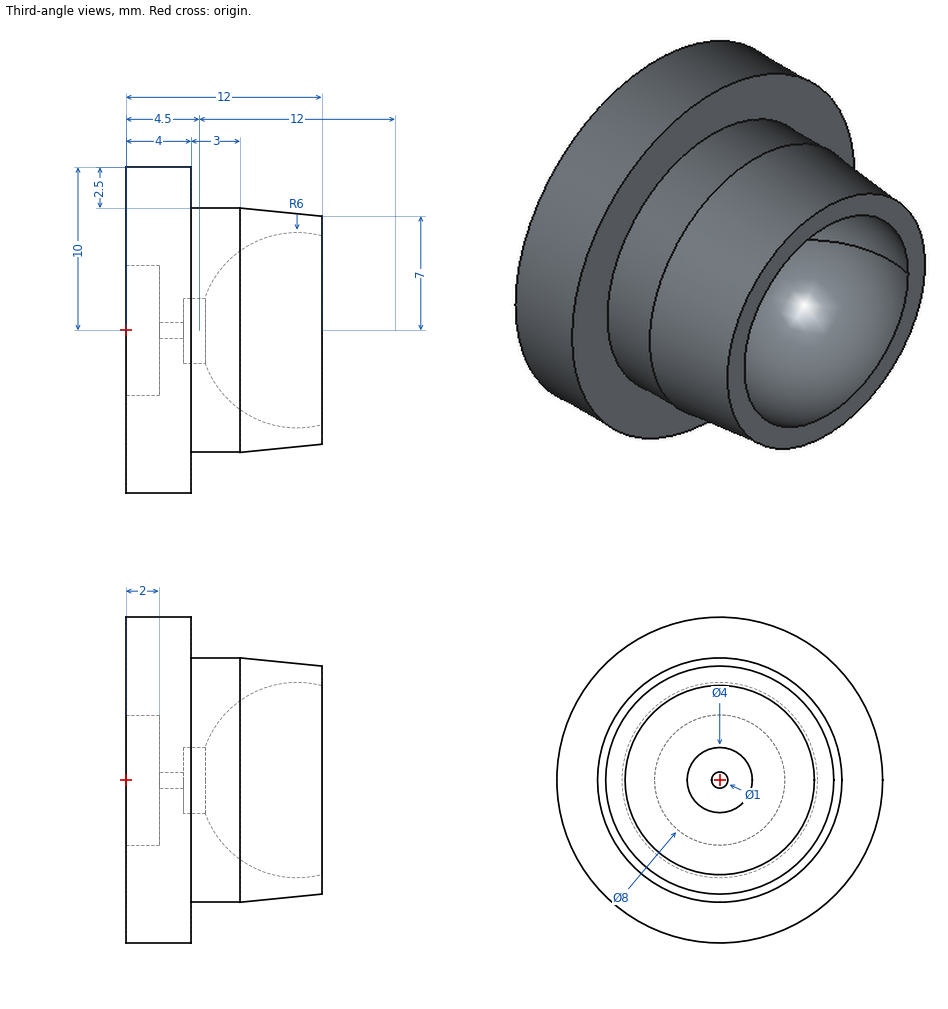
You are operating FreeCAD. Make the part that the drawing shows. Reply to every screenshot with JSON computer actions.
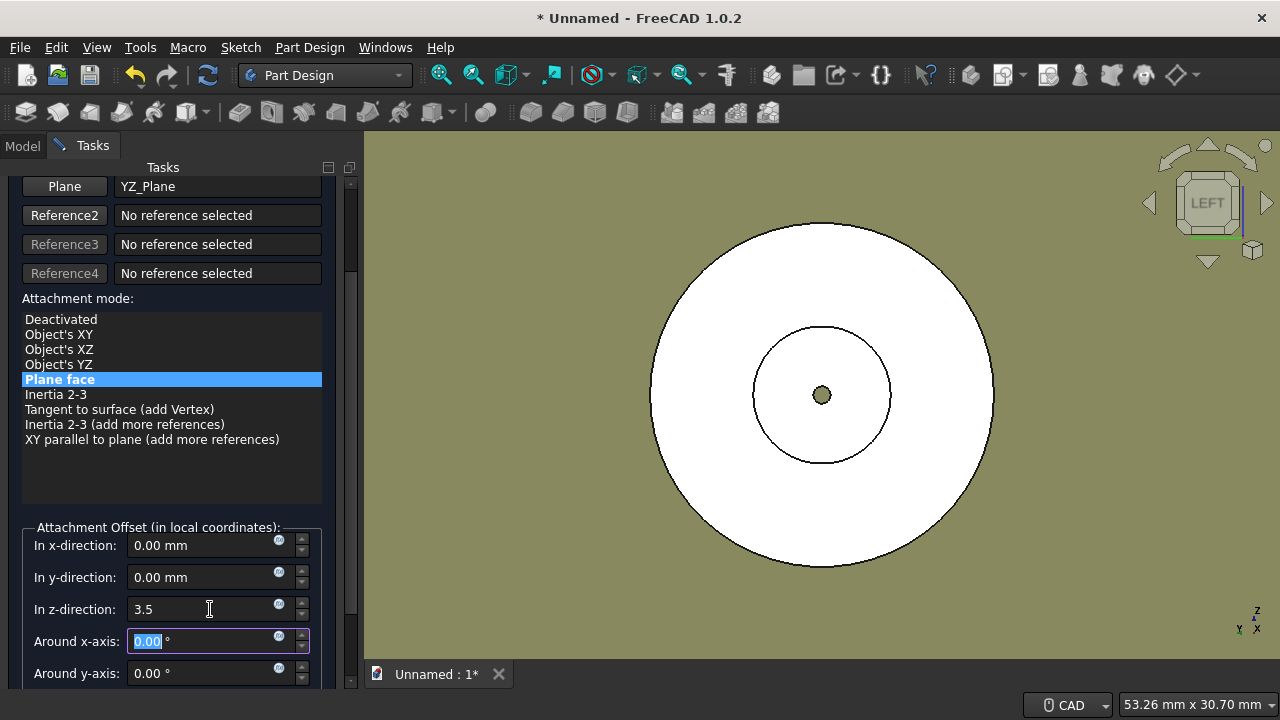
{"action": "scroll", "coordinate": [351, 432], "scroll_direction": "up", "scroll_amount": 3}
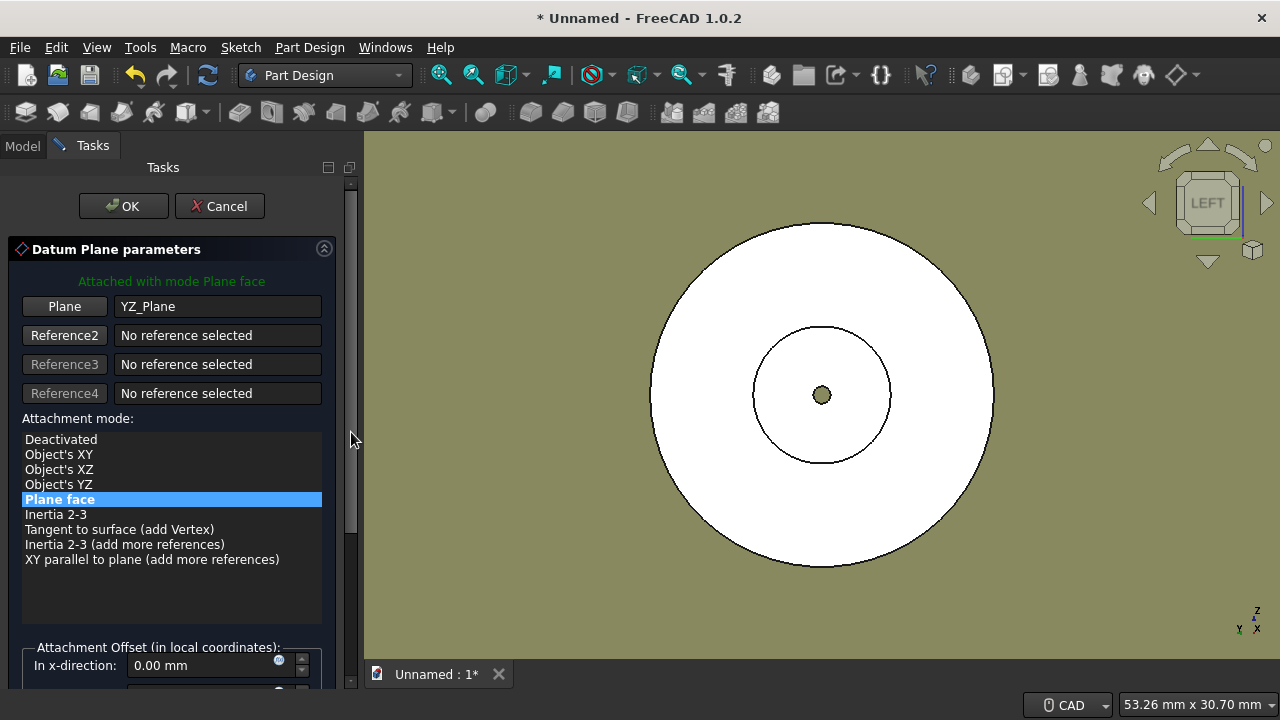
{"action": "left_click", "coordinate": [124, 206]}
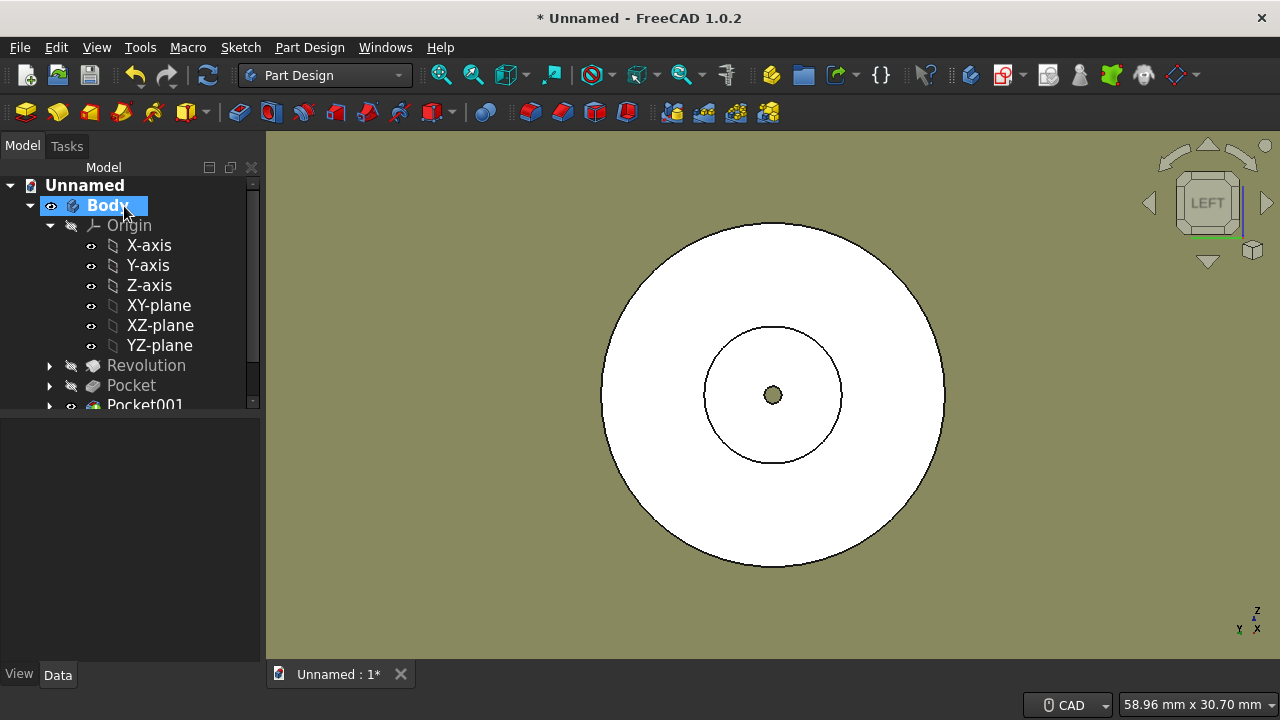
{"action": "scroll", "coordinate": [100, 301], "scroll_direction": "down", "scroll_amount": 3}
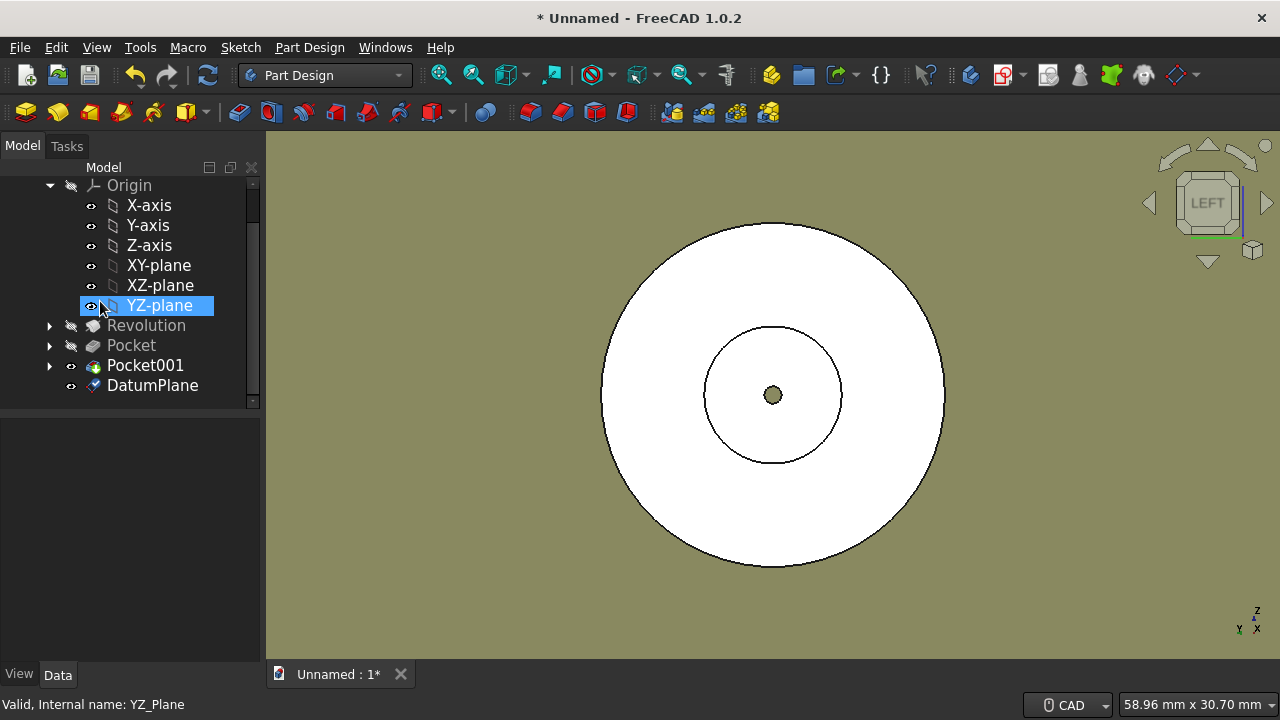
{"action": "left_click", "coordinate": [116, 386]}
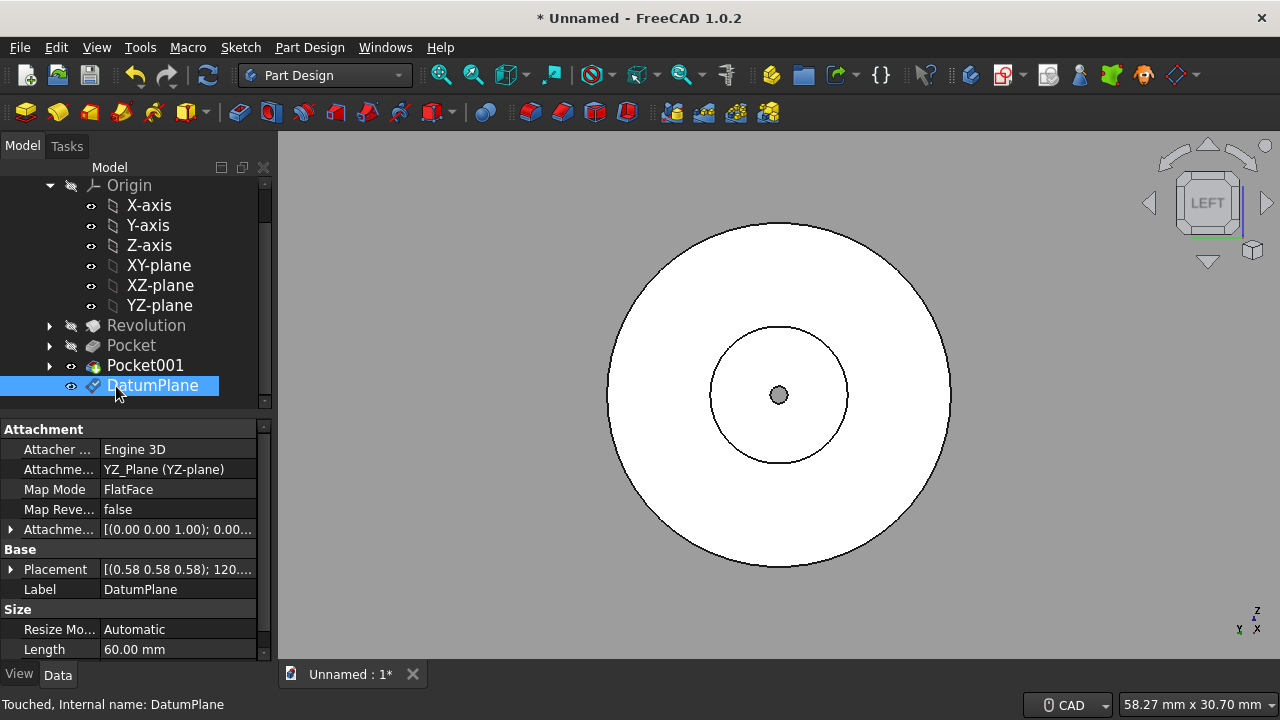
{"action": "left_click", "coordinate": [1004, 76]}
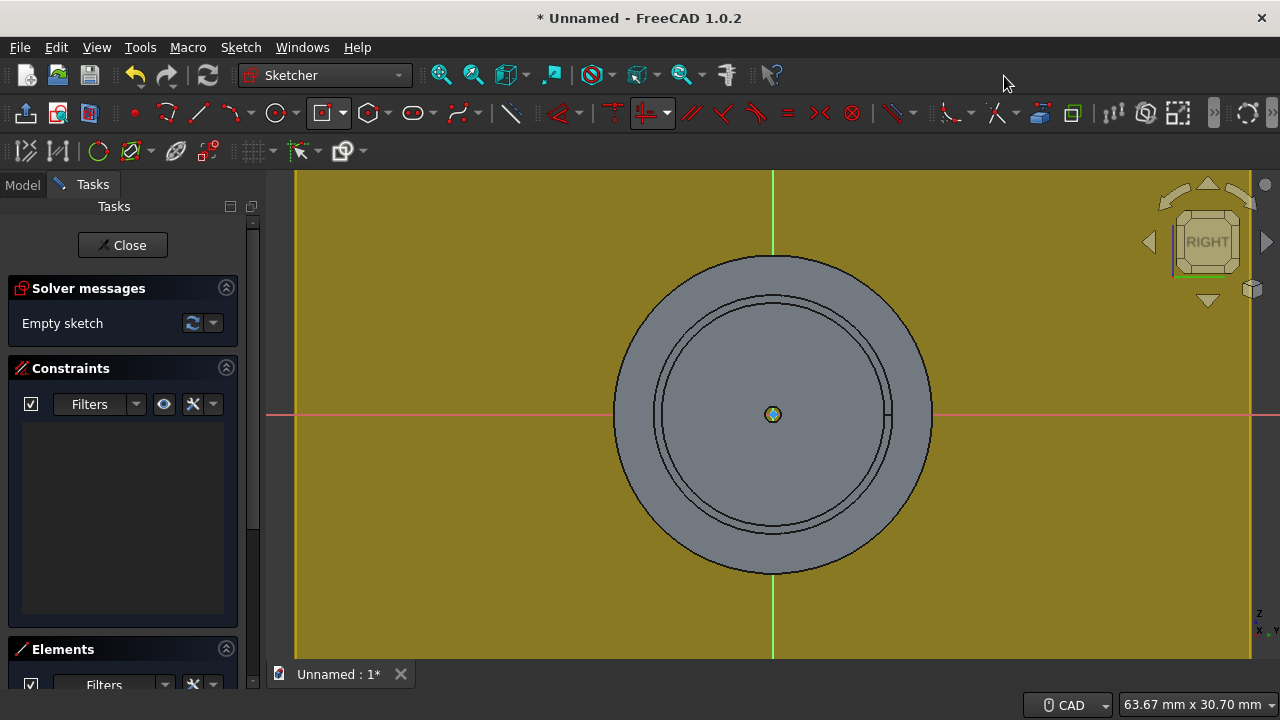
{"action": "left_click", "coordinate": [90, 114]}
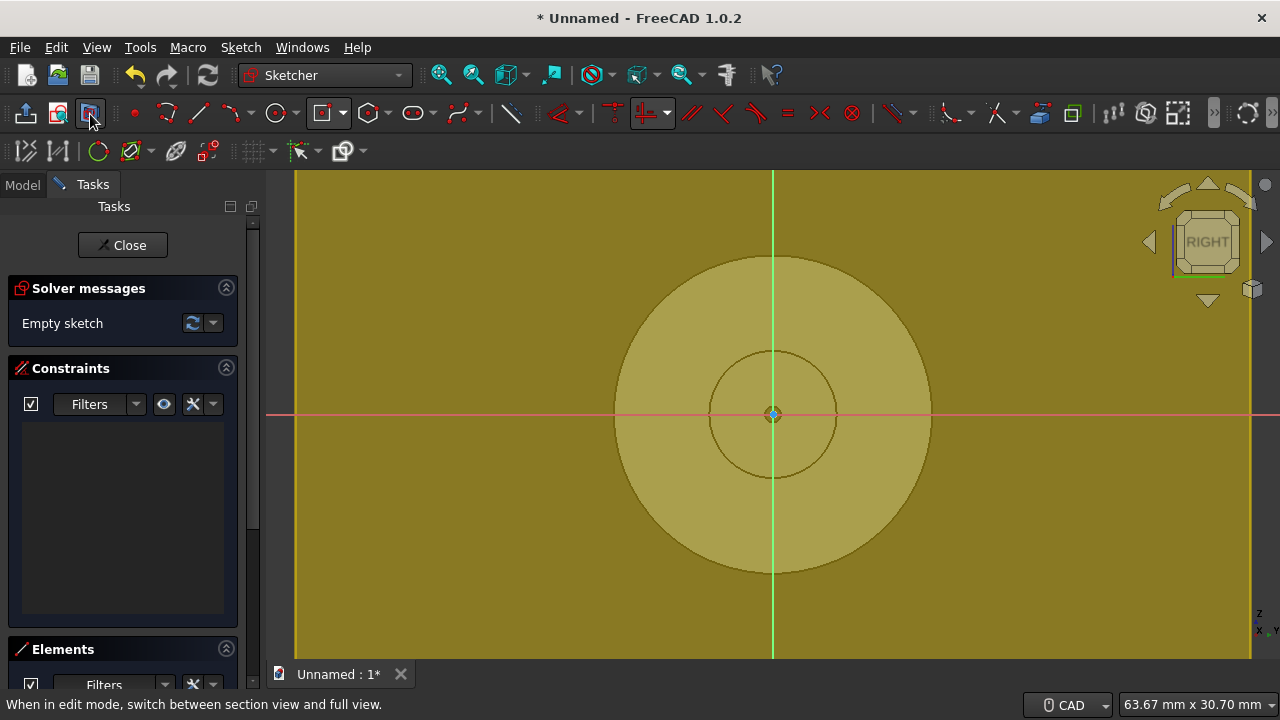
{"action": "scroll", "coordinate": [790, 415], "scroll_direction": "up", "scroll_amount": 8}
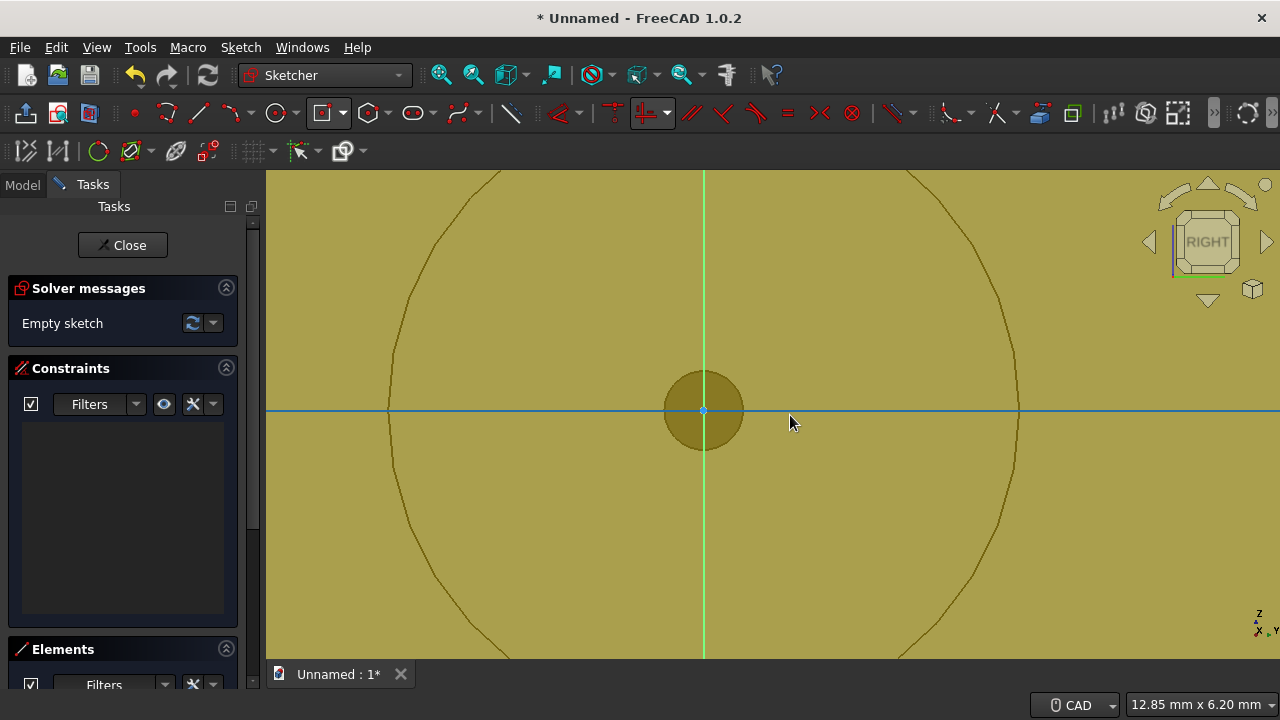
{"action": "left_click", "coordinate": [276, 114]}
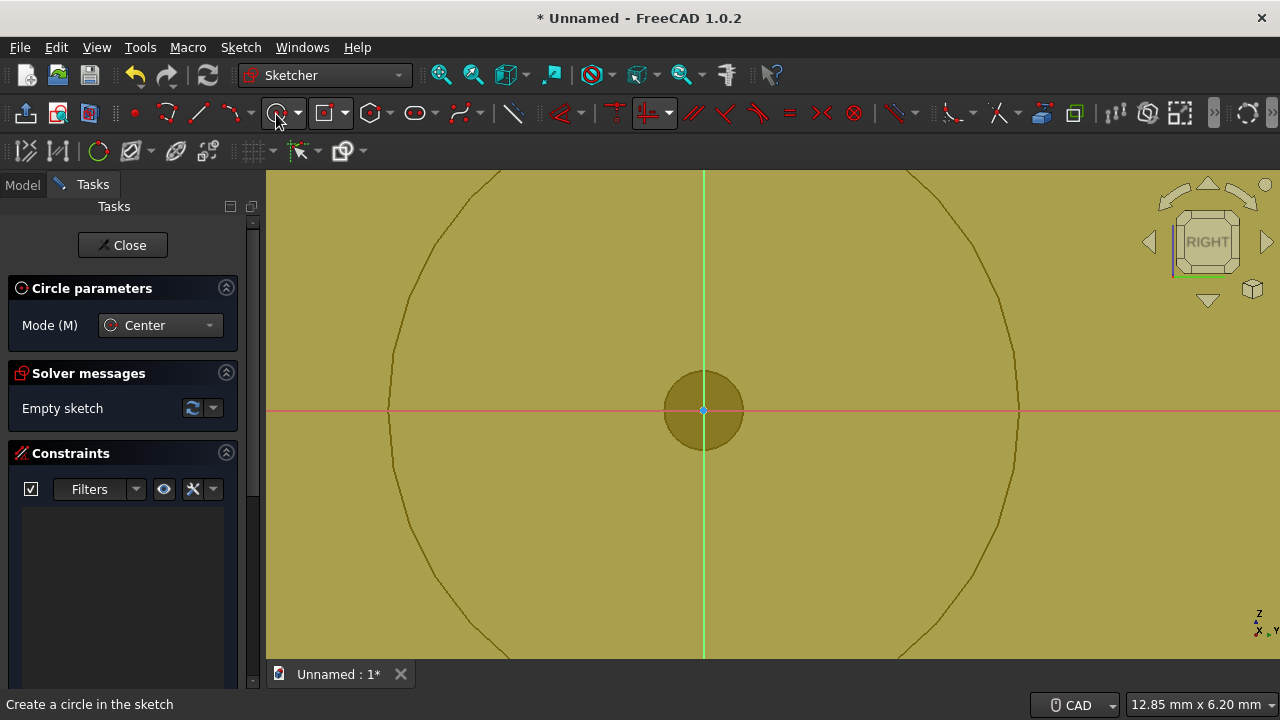
{"action": "left_click", "coordinate": [704, 411]}
{"action": "mouse_move", "coordinate": [815, 299]}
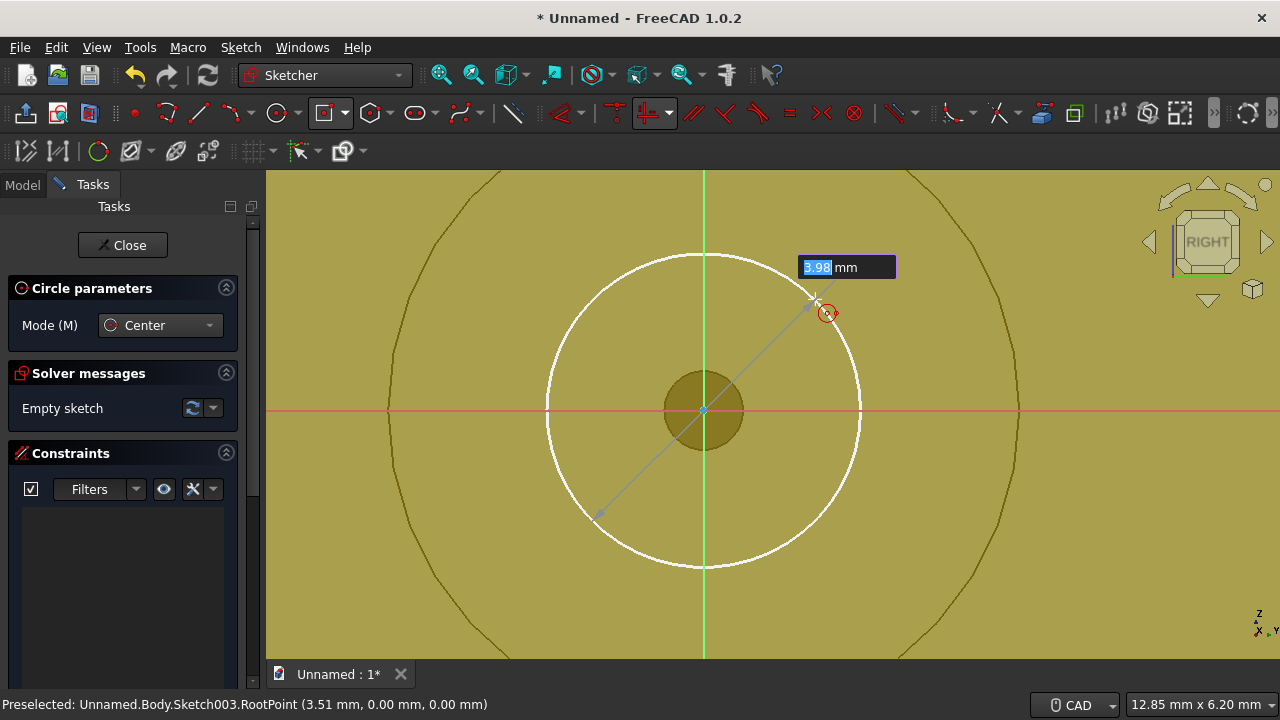
{"action": "type", "text": "4"}
{"action": "key", "text": "Return"}
{"action": "key", "text": "Escape"}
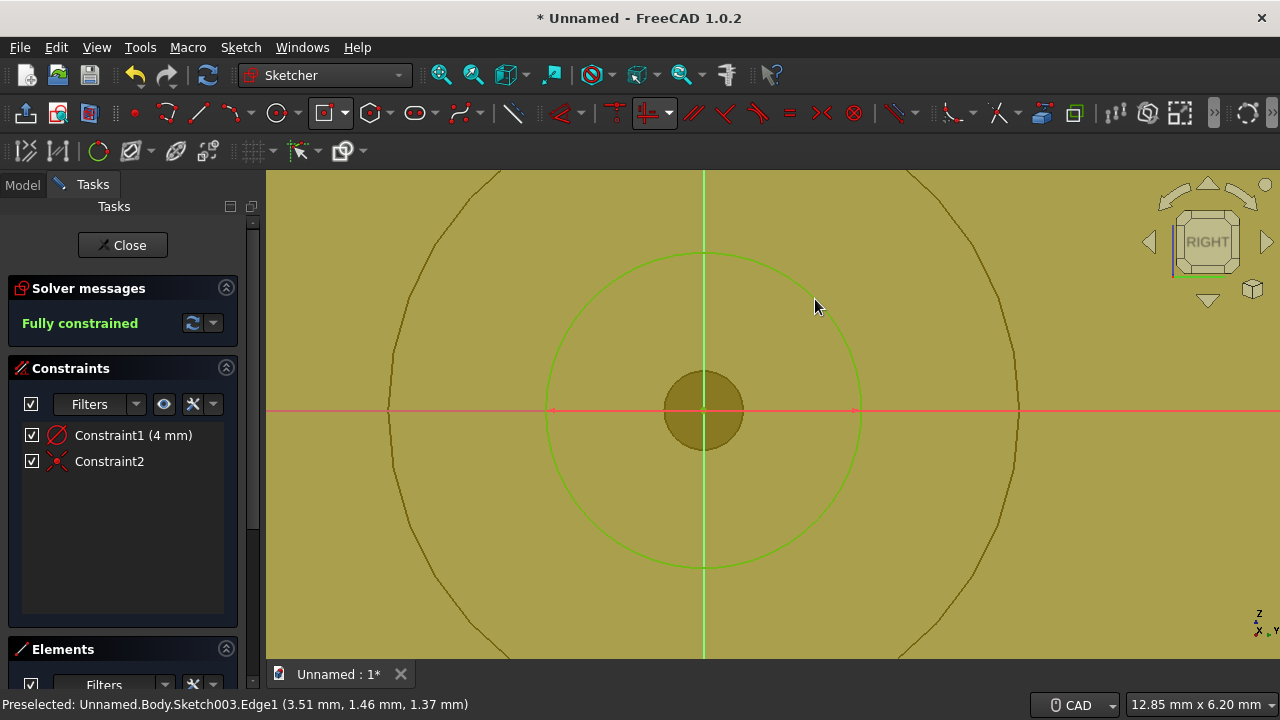
{"action": "left_click", "coordinate": [123, 245]}